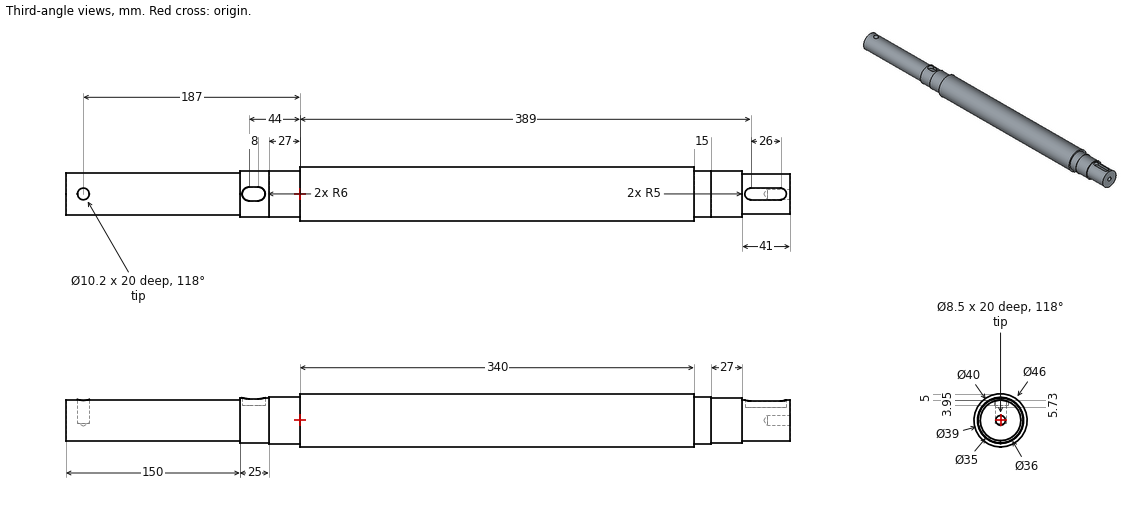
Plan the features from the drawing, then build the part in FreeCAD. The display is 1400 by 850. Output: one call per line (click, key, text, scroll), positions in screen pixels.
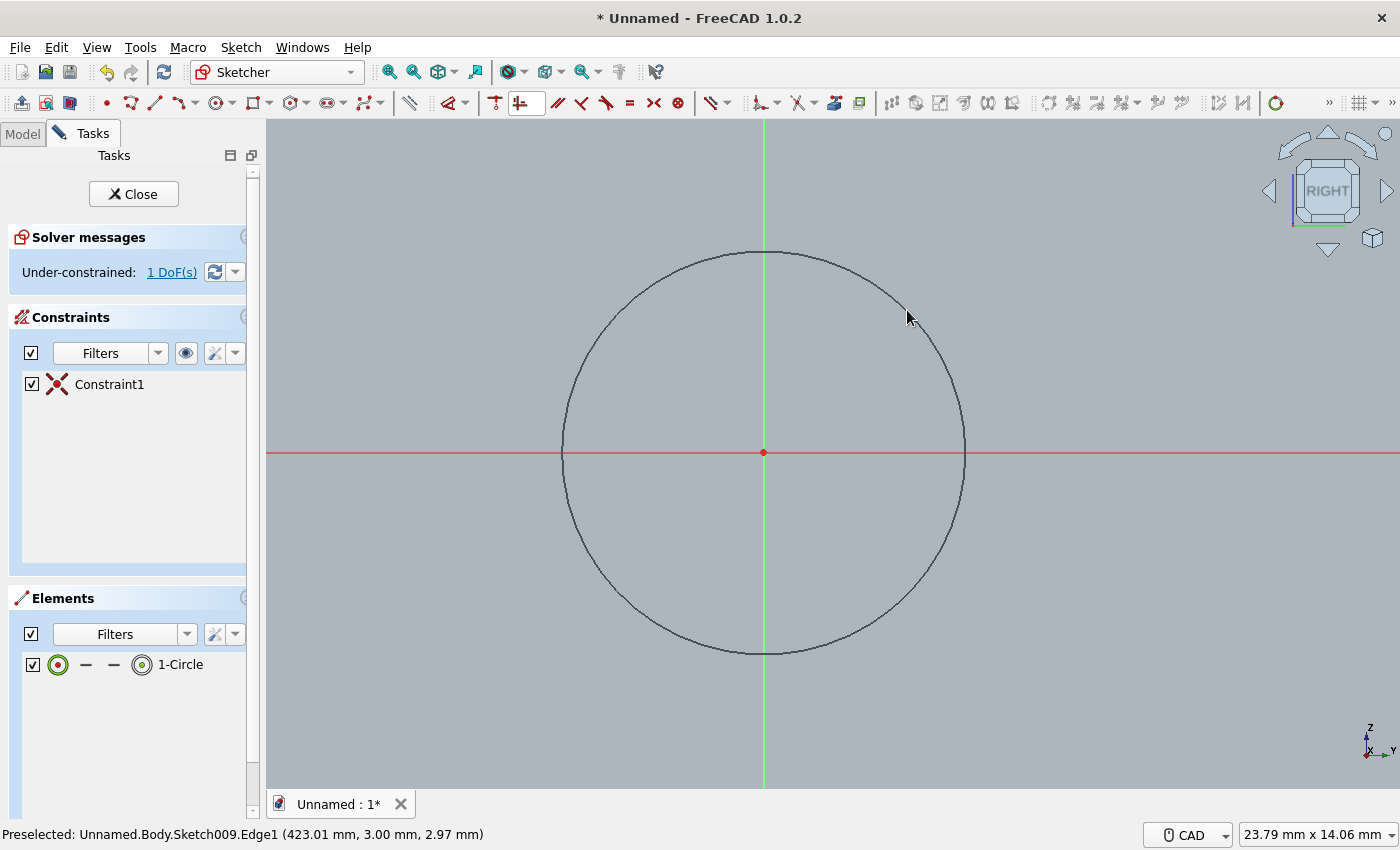
click(448, 104)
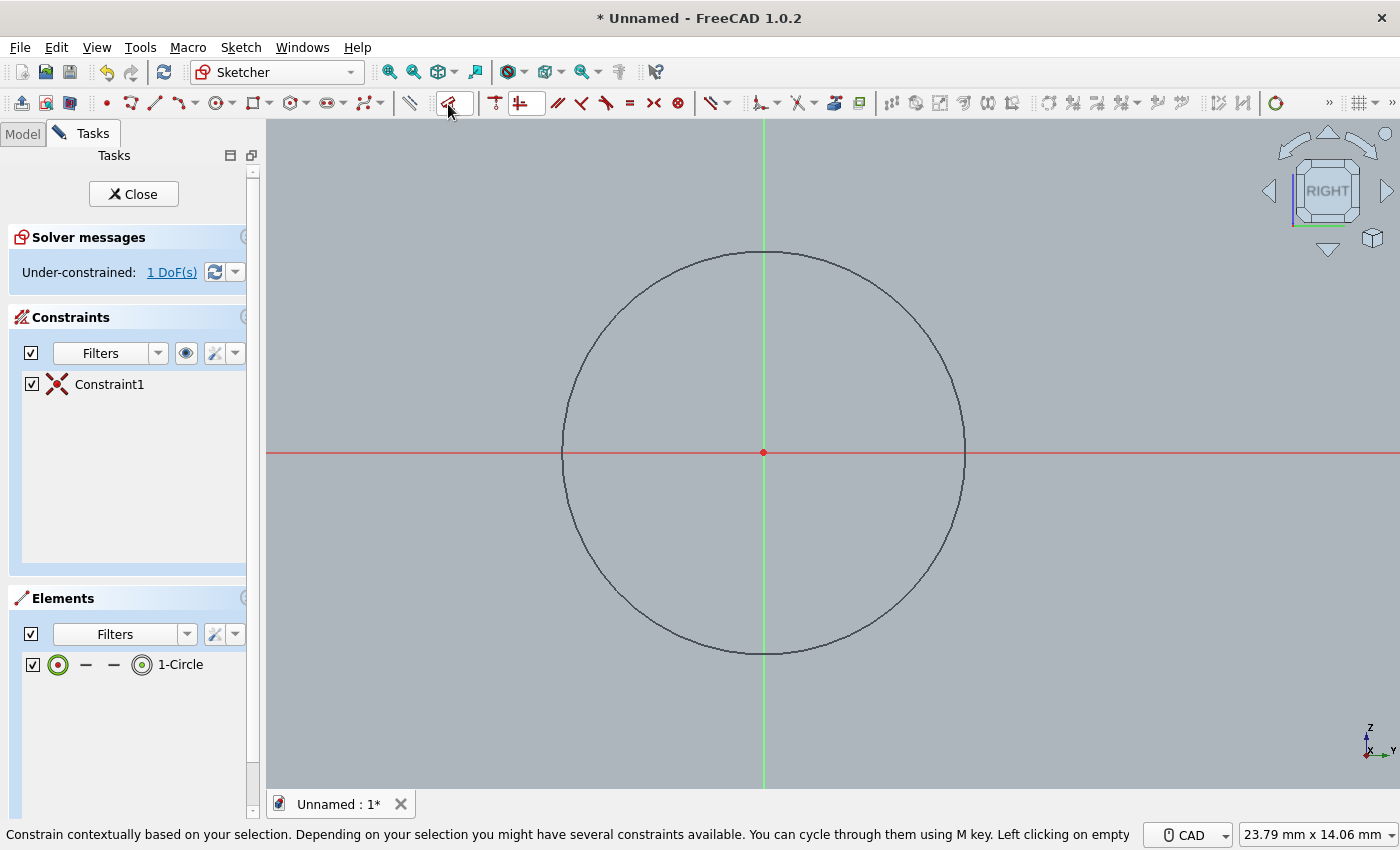
click(906, 310)
click(929, 287)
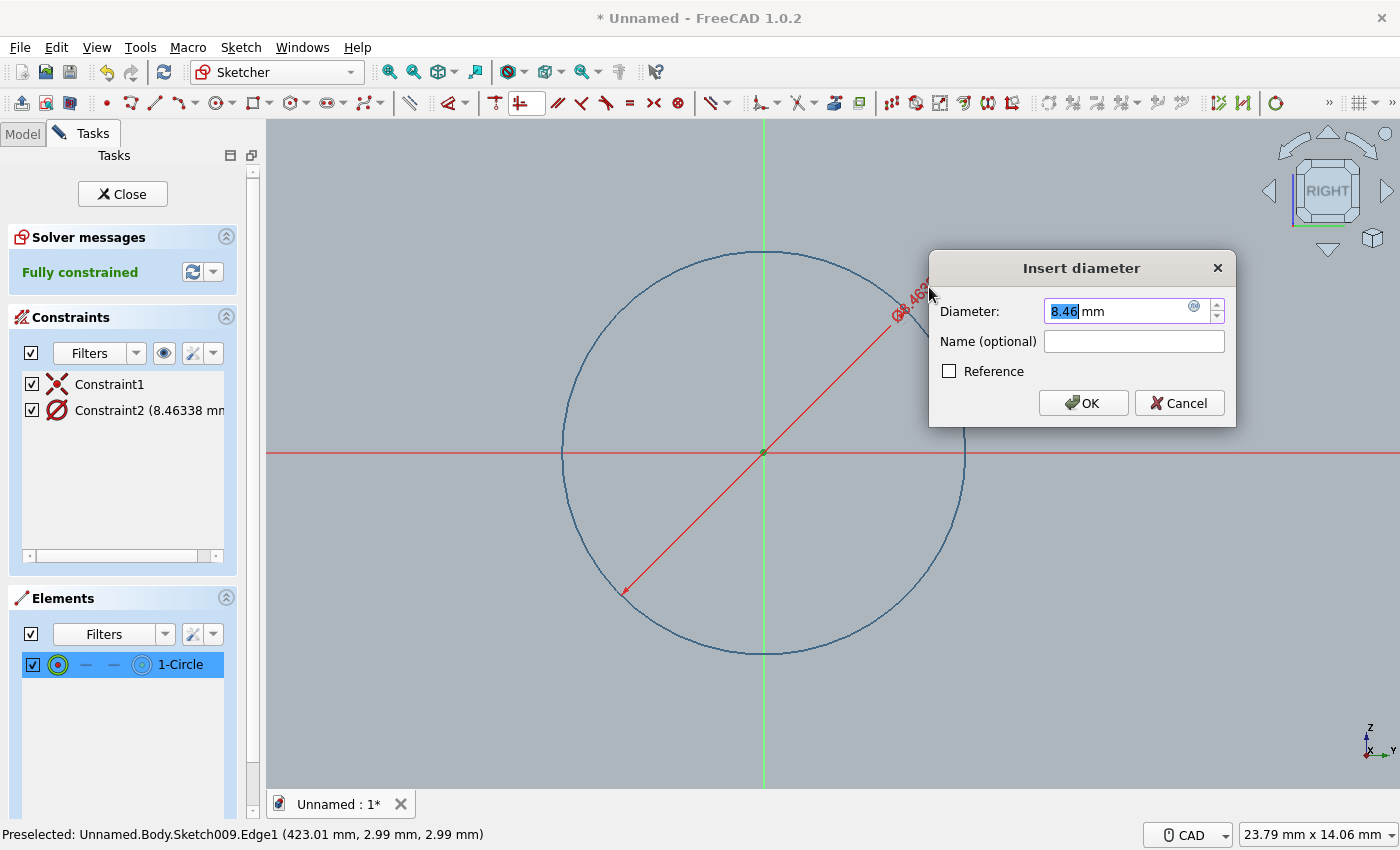
text(8.5)
key(Return)
key(Escape)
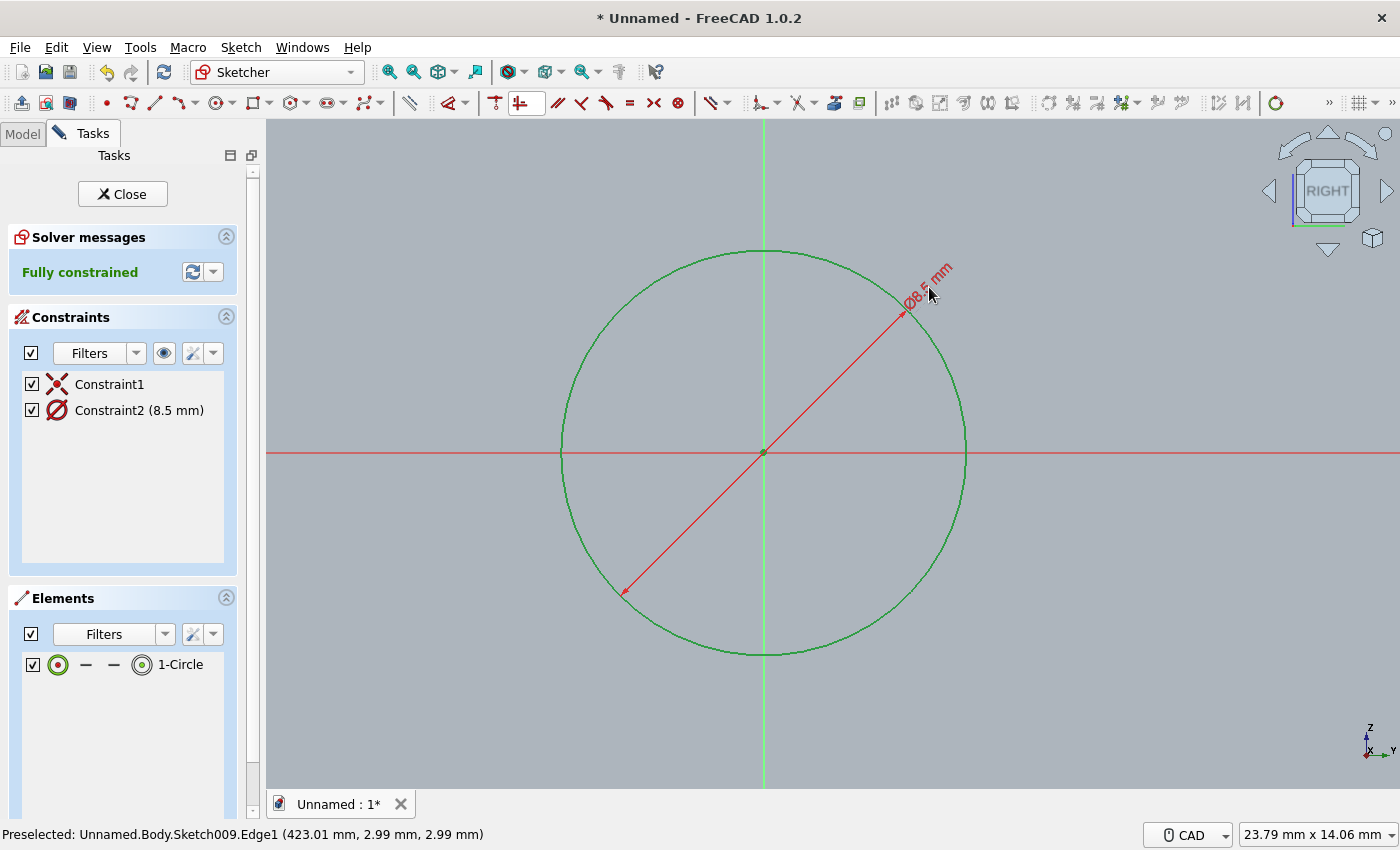
click(123, 194)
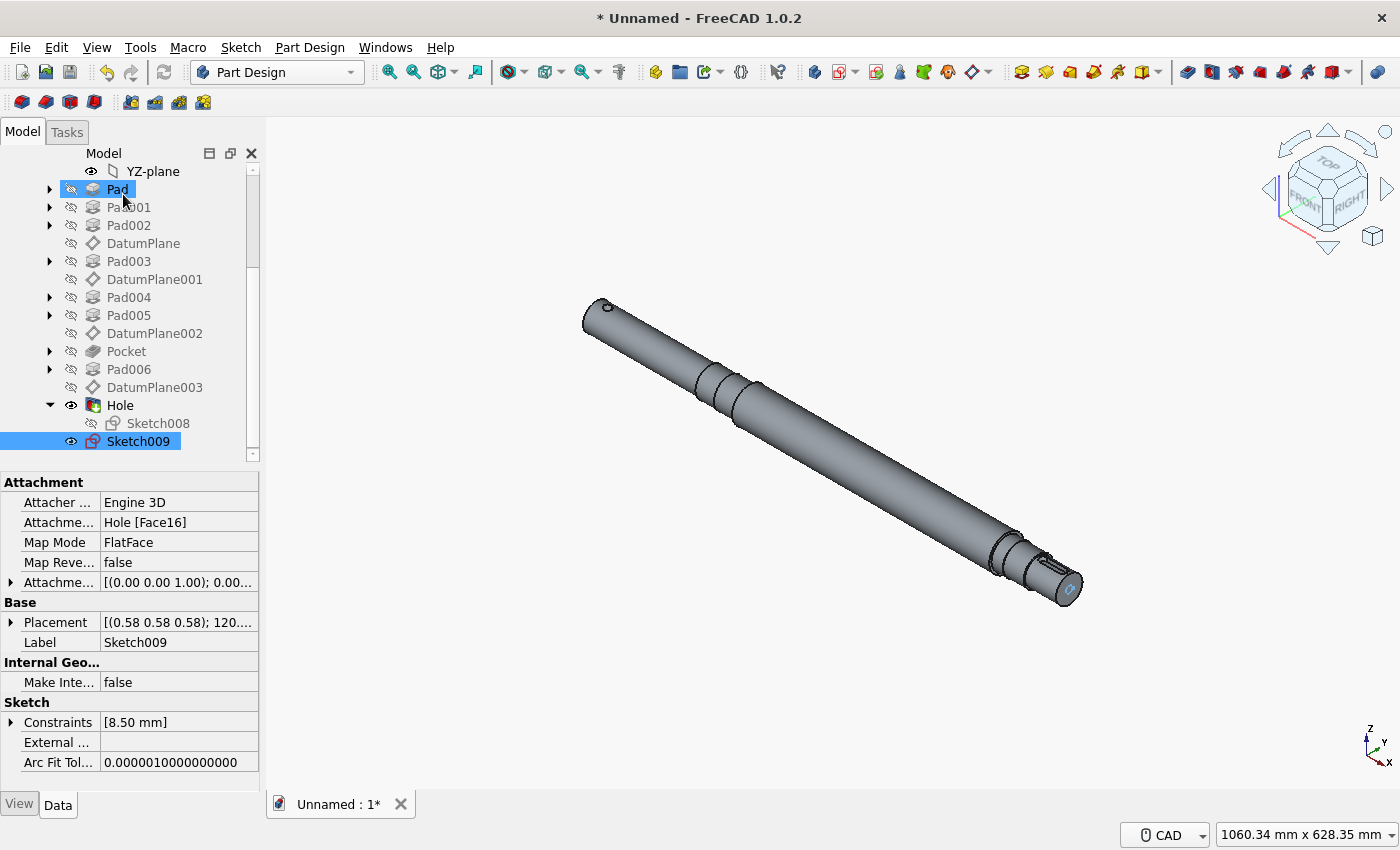
click(1212, 72)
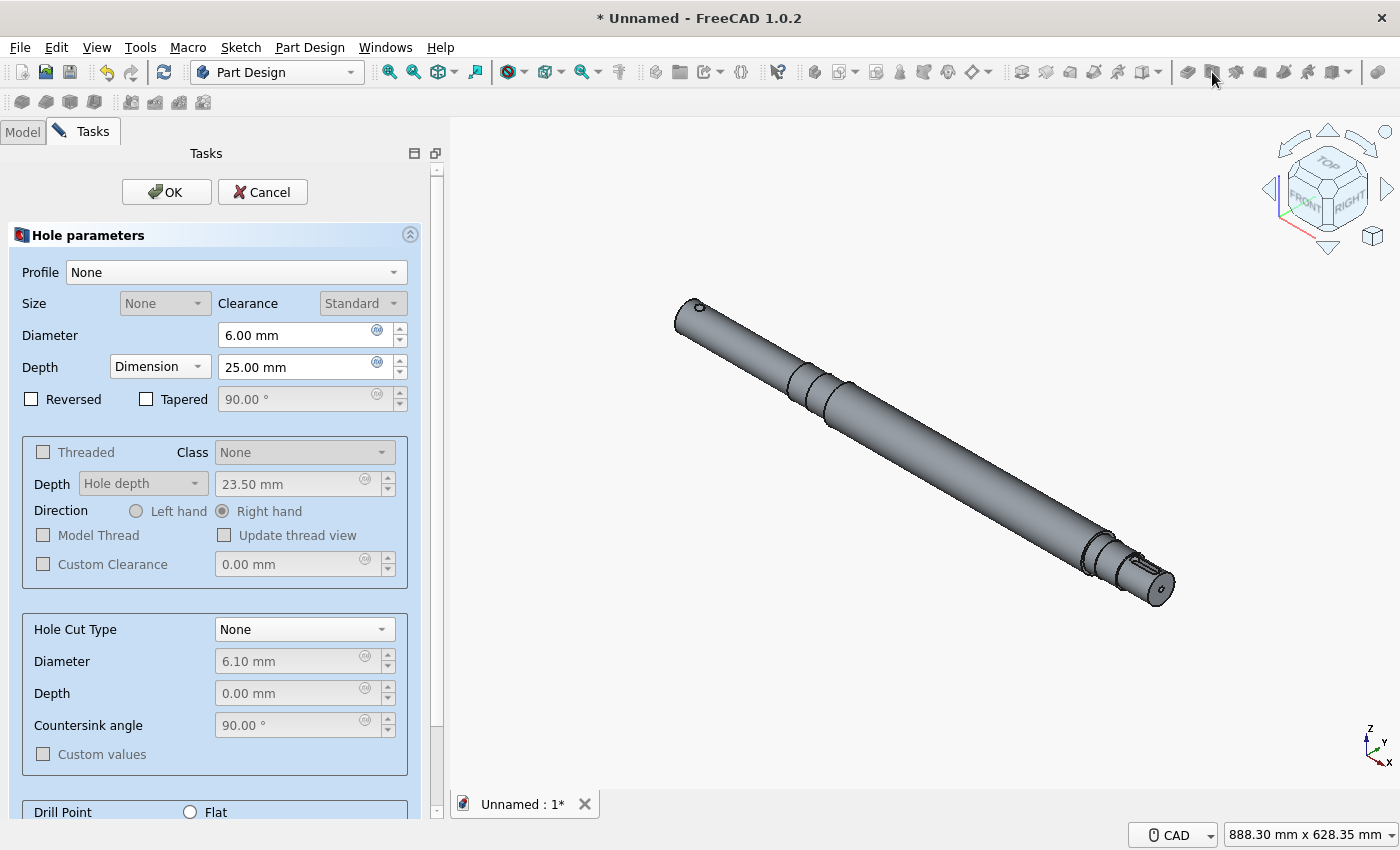
triple_click(305, 335)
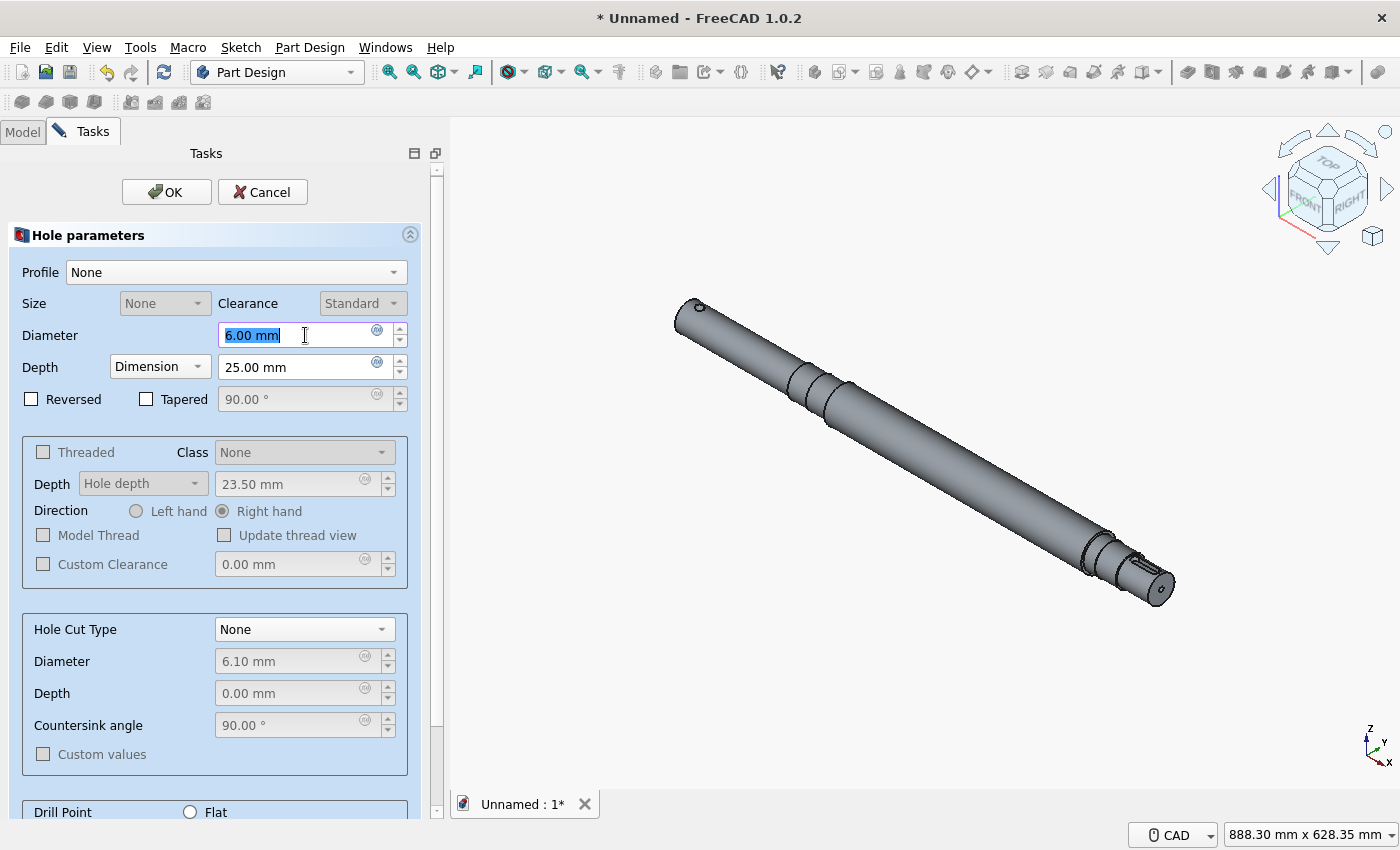
text(8.5)
key(Tab)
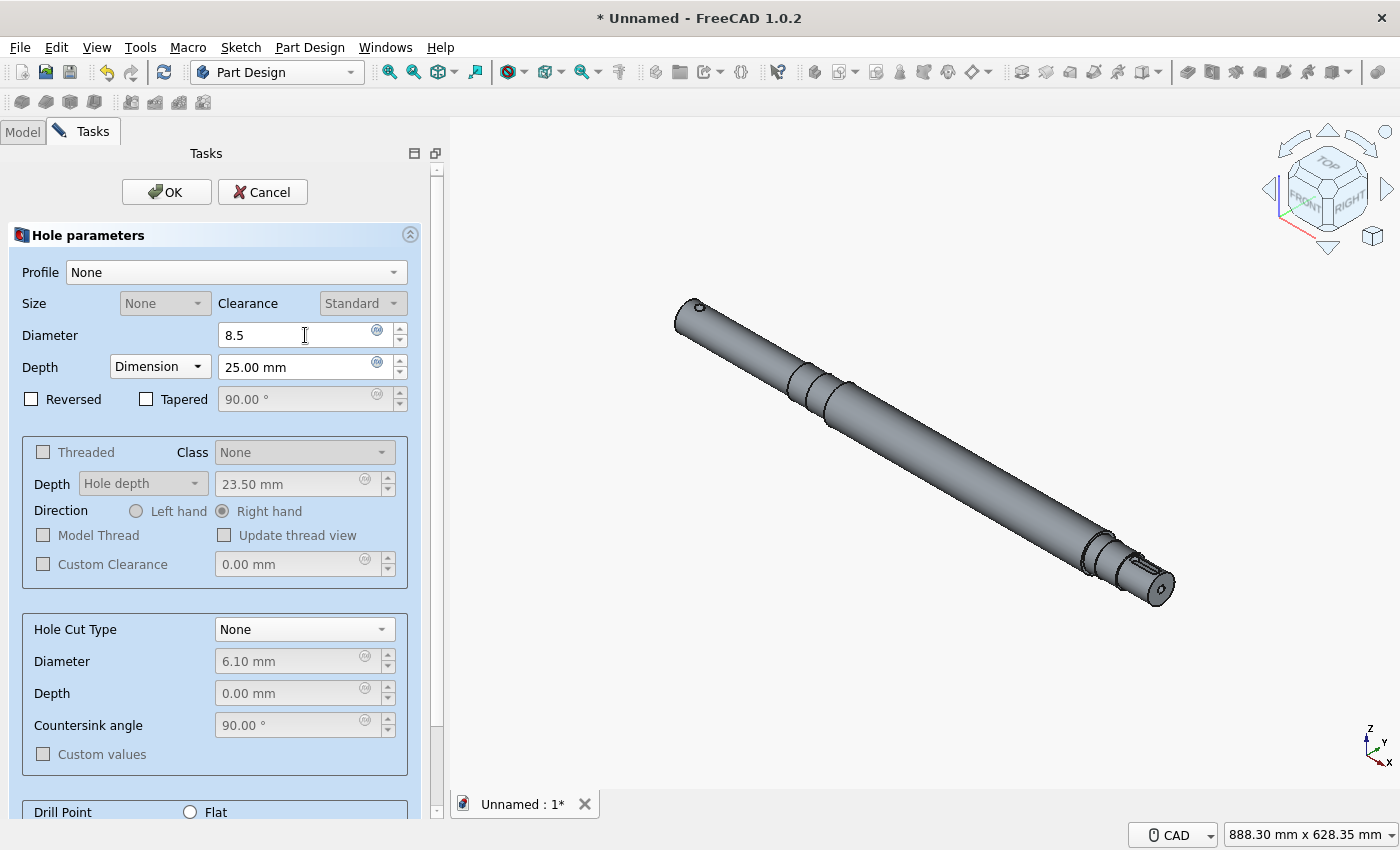
triple_click(305, 367)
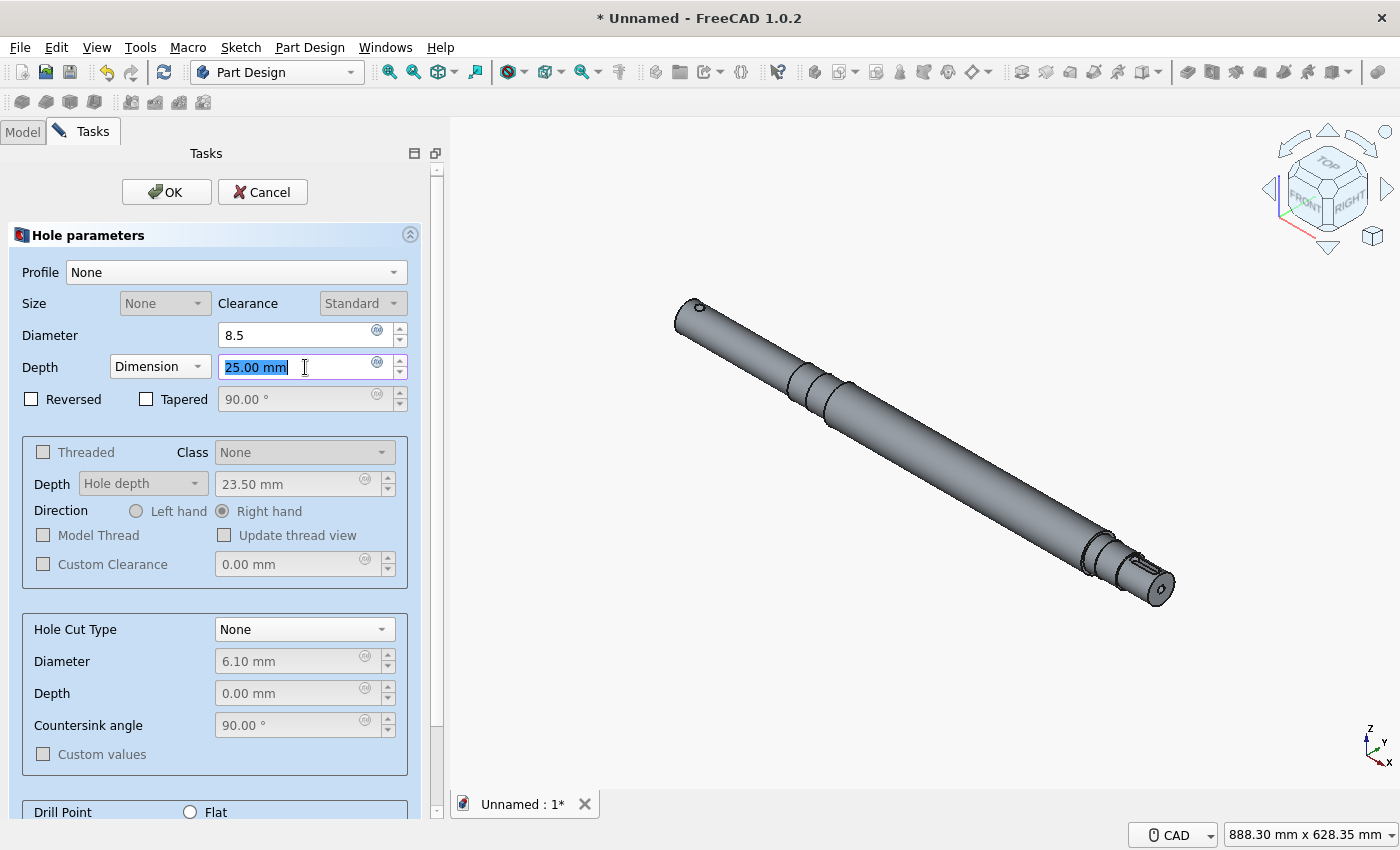
text(20)
key(Tab)